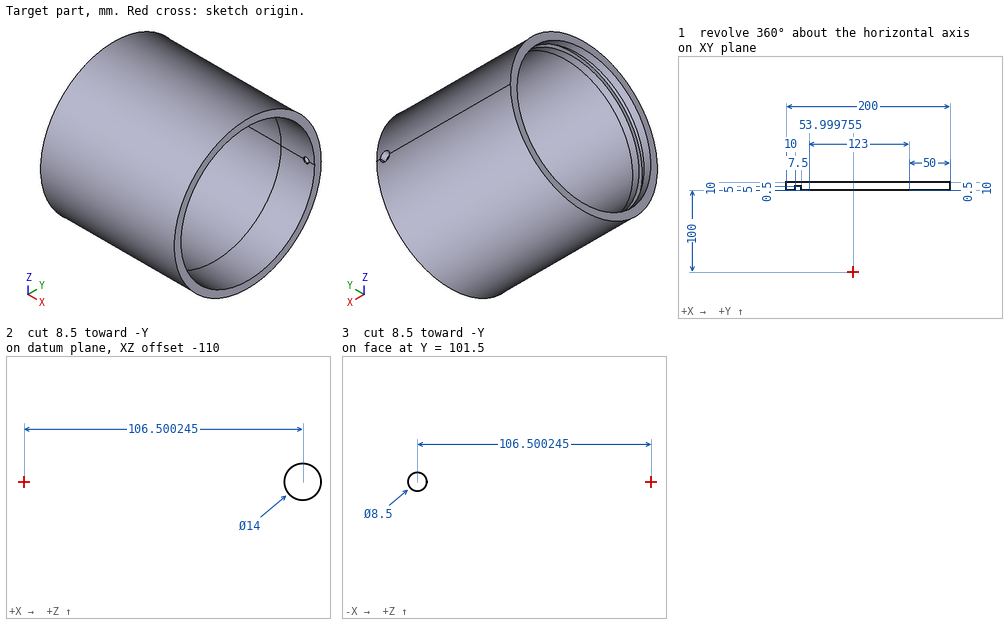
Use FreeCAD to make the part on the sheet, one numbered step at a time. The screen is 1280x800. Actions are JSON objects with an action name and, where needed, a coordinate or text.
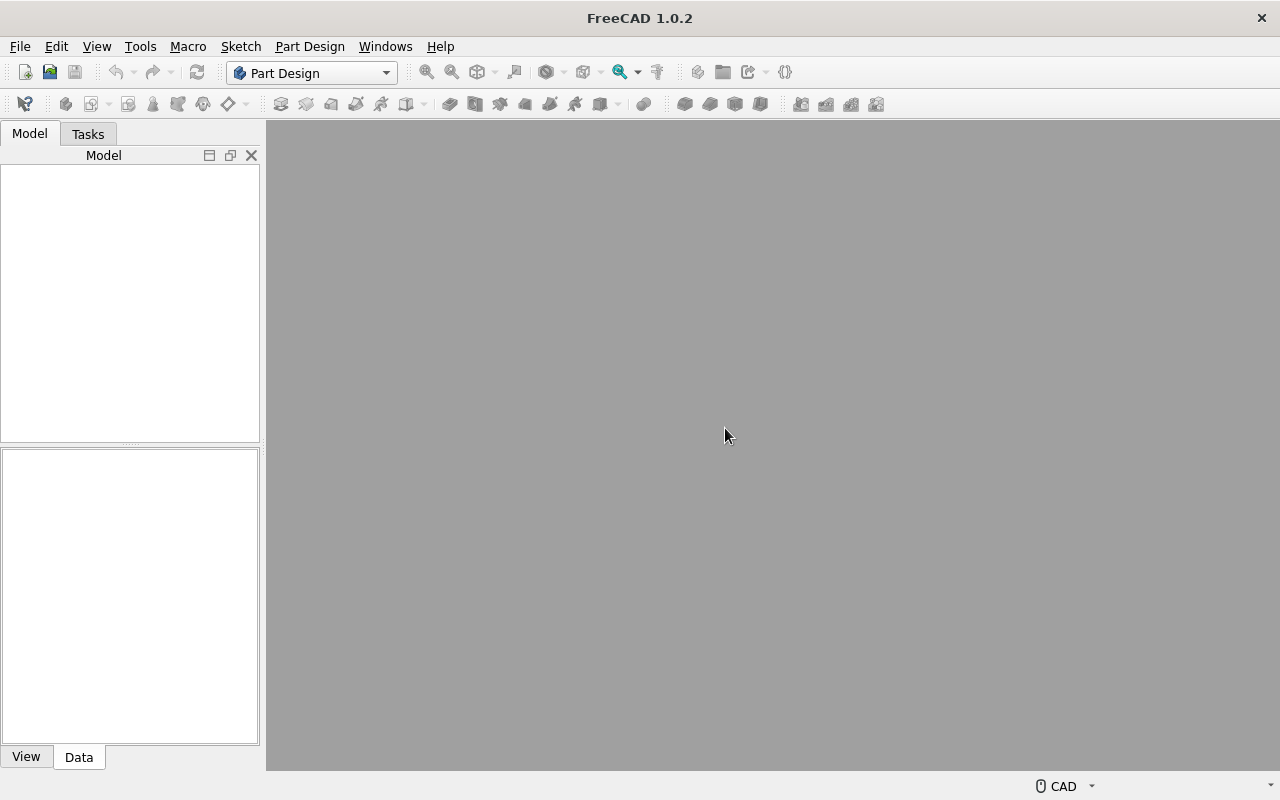
{"action": "key", "text": "ctrl+n"}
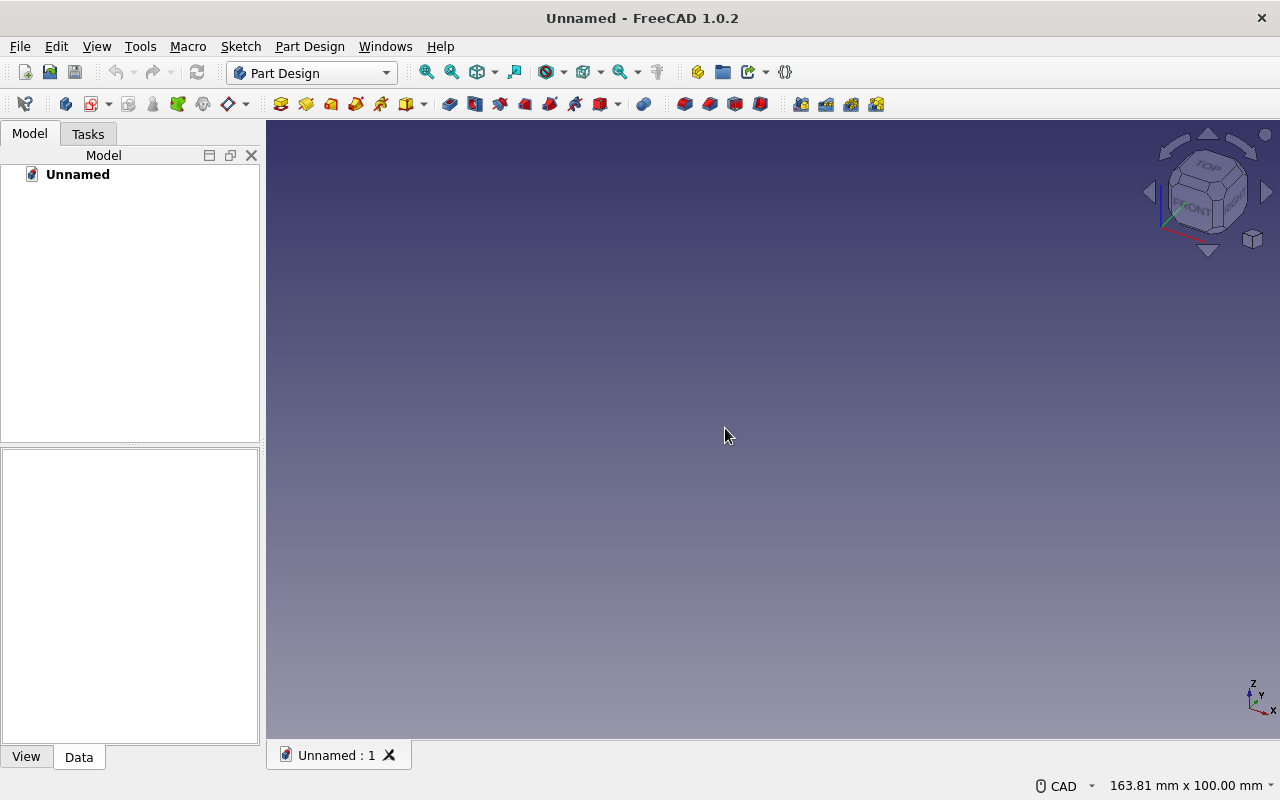
{"action": "left_click", "coordinate": [90, 104]}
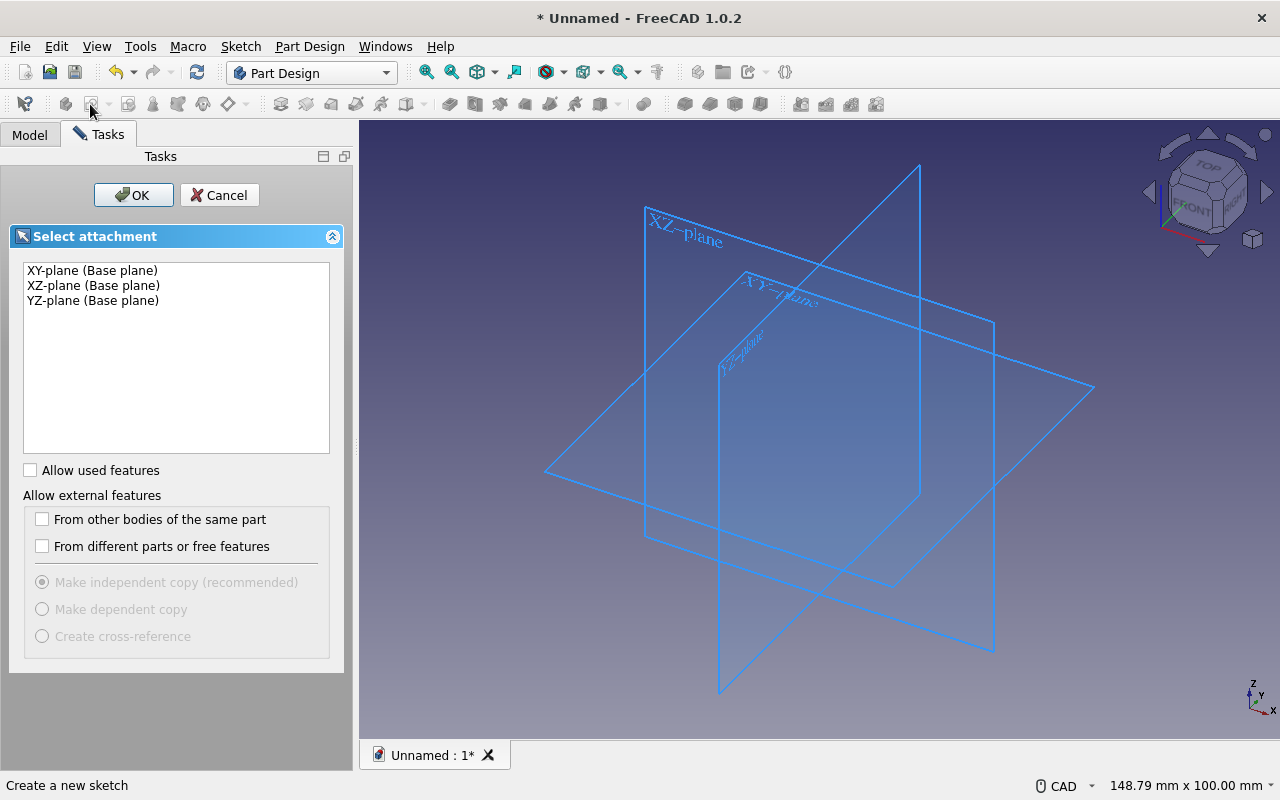
{"action": "left_click", "coordinate": [84, 270]}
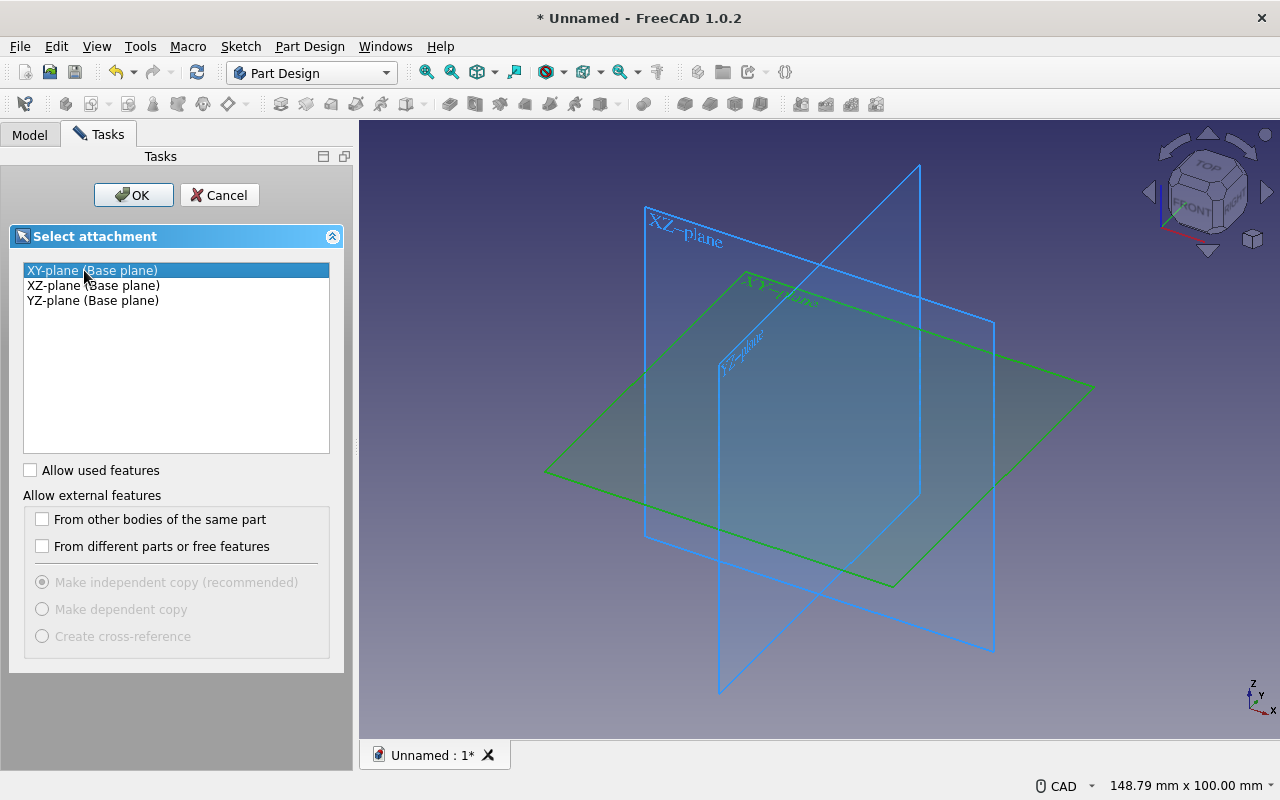
{"action": "left_click", "coordinate": [134, 195]}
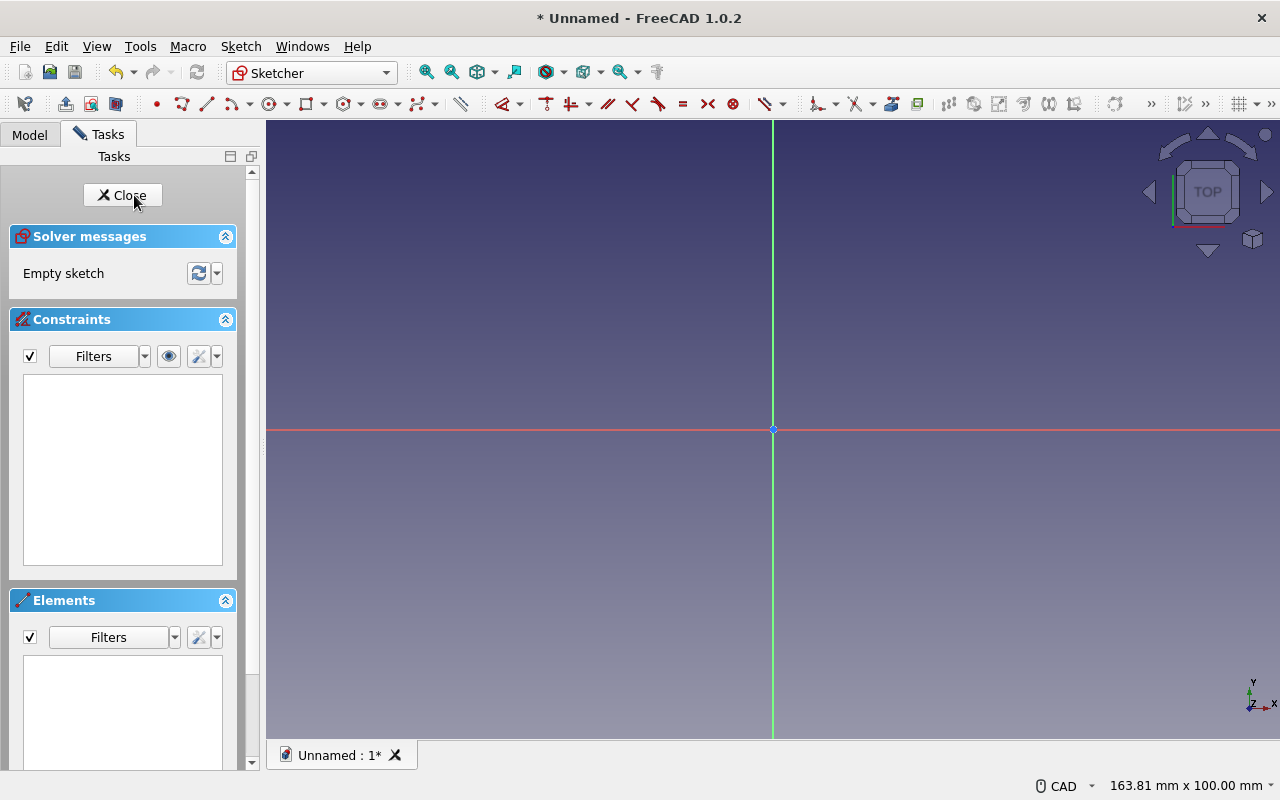
{"action": "scroll", "coordinate": [553, 707], "scroll_direction": "down", "scroll_amount": 4}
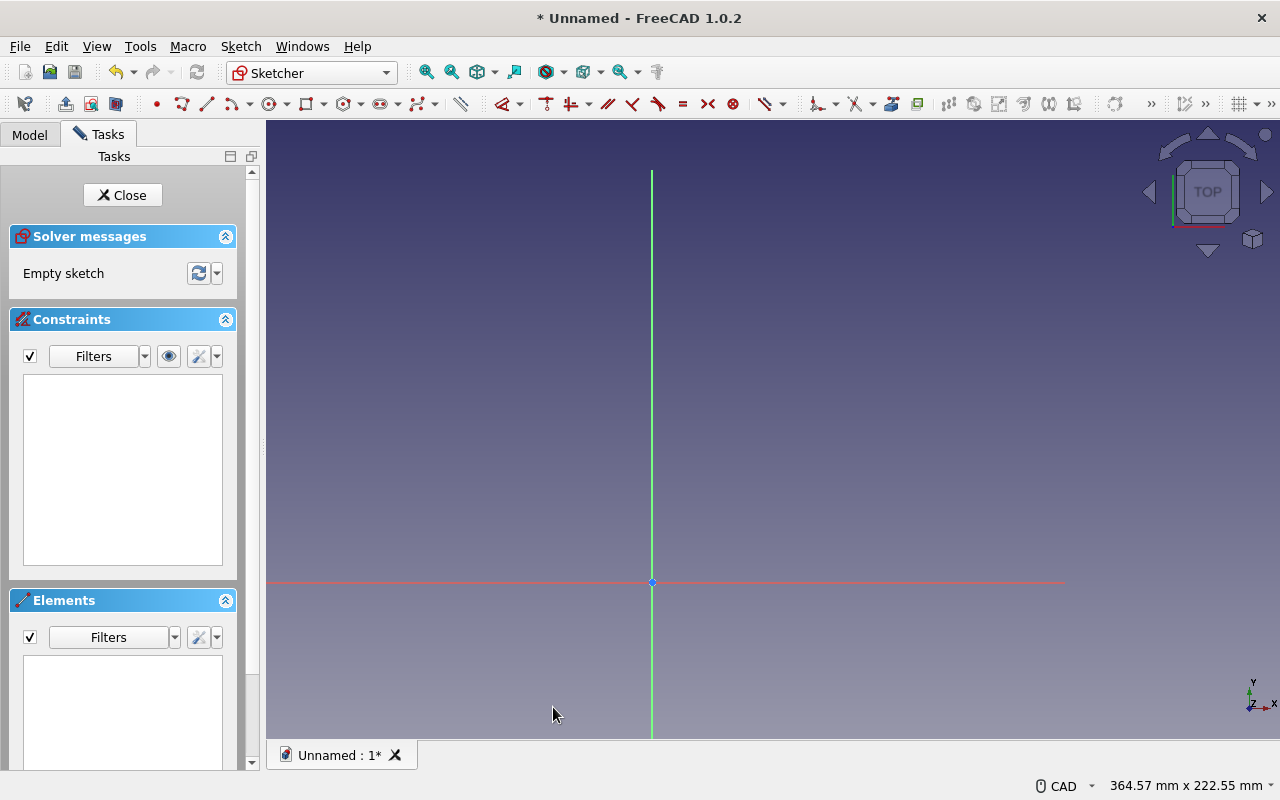
{"action": "key", "text": "g m"}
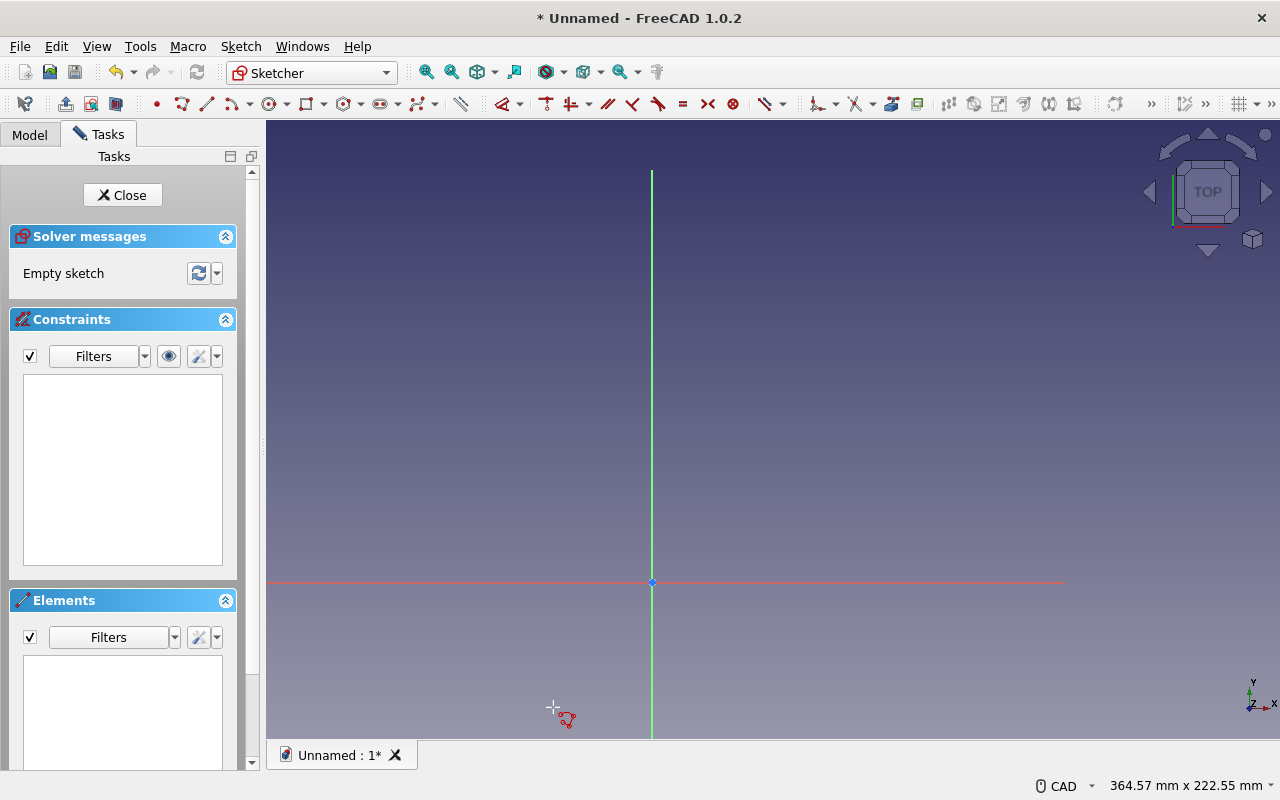
{"action": "left_click", "coordinate": [502, 305]}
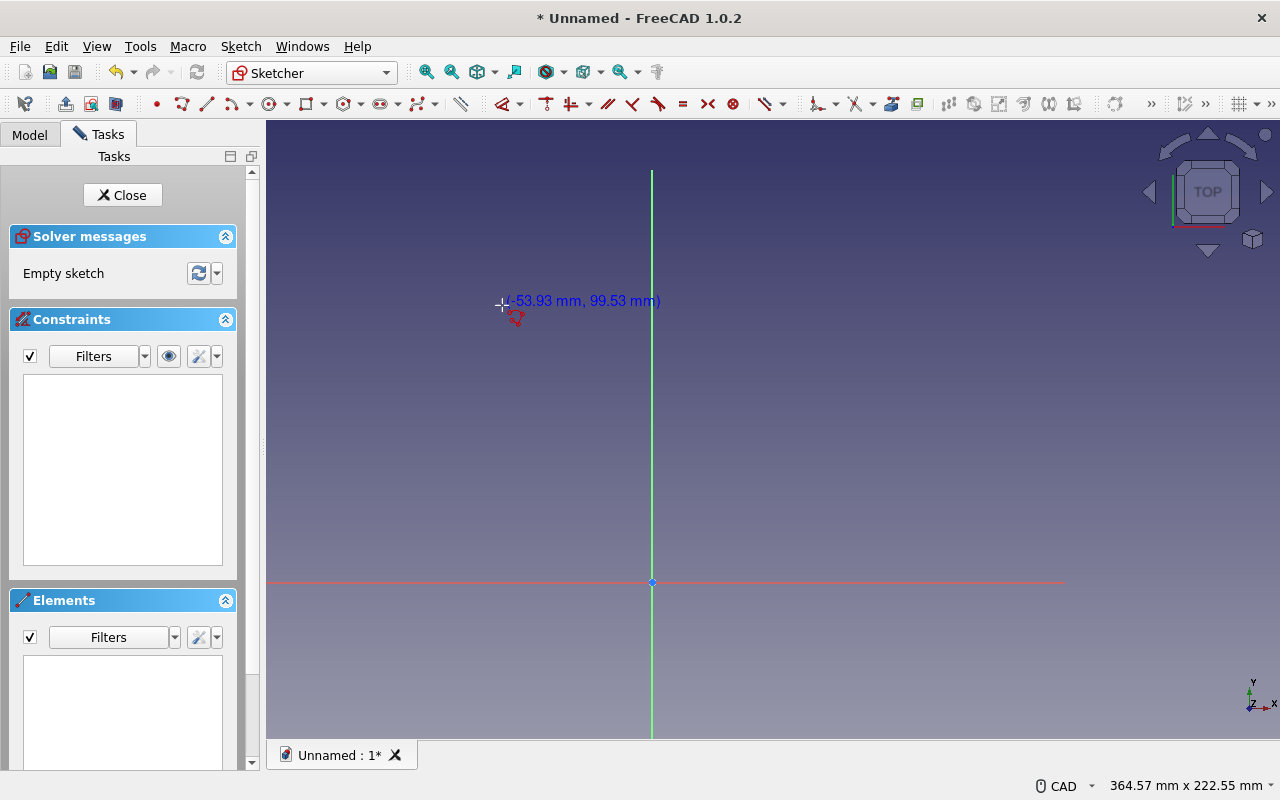
{"action": "scroll", "coordinate": [502, 303], "scroll_direction": "up", "scroll_amount": 13}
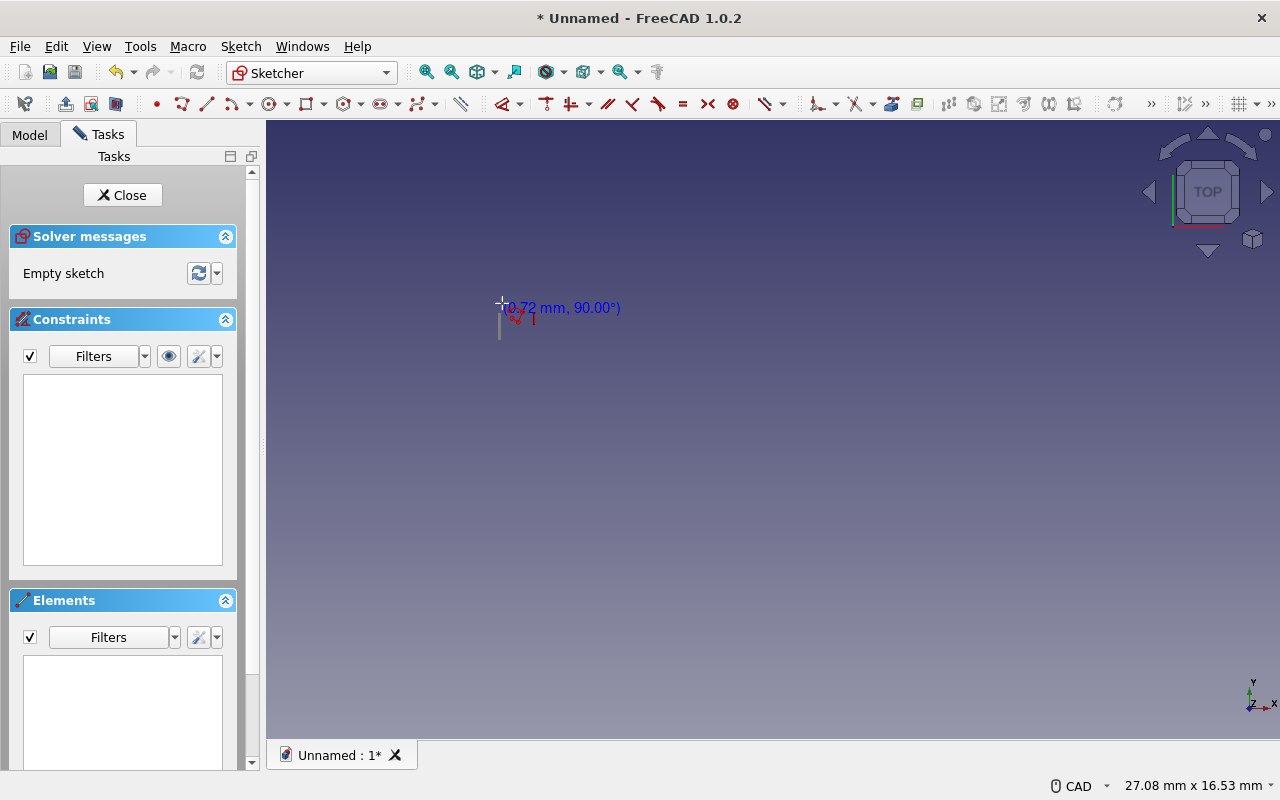
{"action": "left_click", "coordinate": [499, 303]}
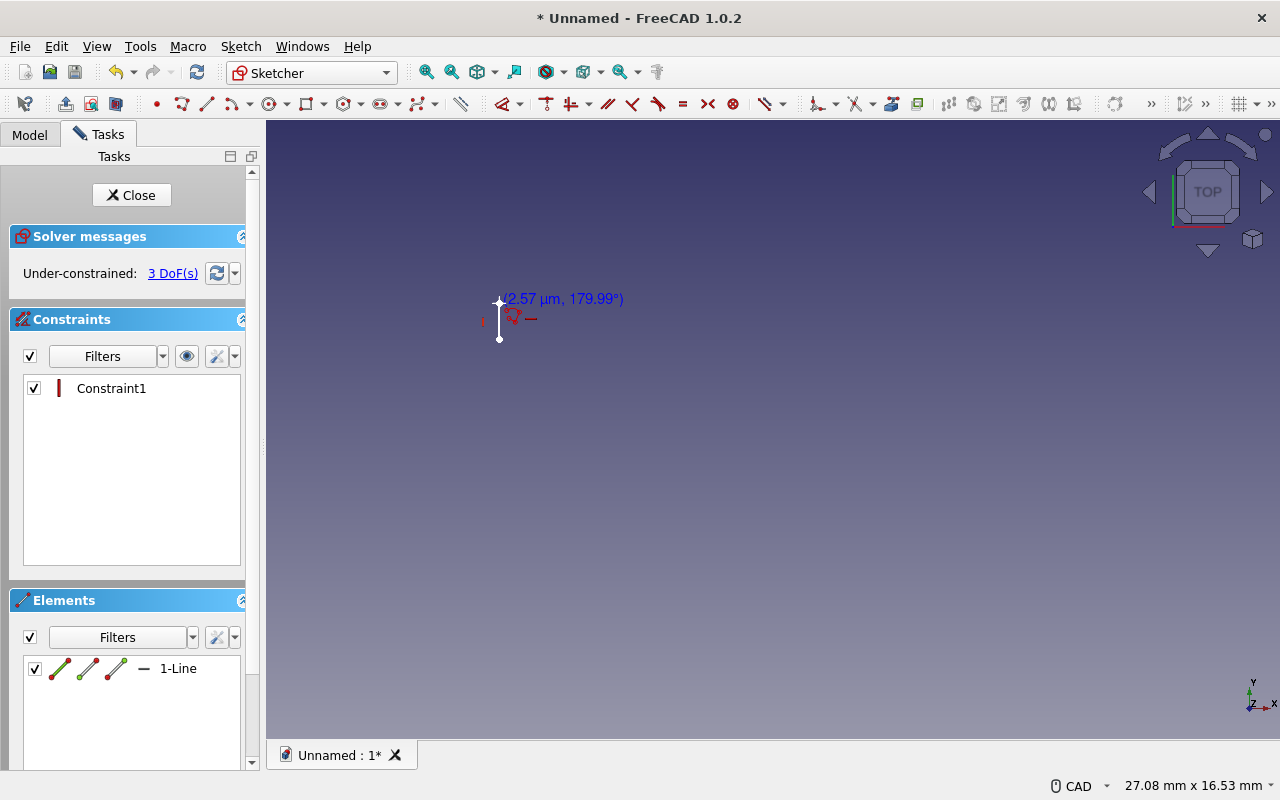
{"action": "scroll", "coordinate": [502, 303], "scroll_direction": "down", "scroll_amount": 13}